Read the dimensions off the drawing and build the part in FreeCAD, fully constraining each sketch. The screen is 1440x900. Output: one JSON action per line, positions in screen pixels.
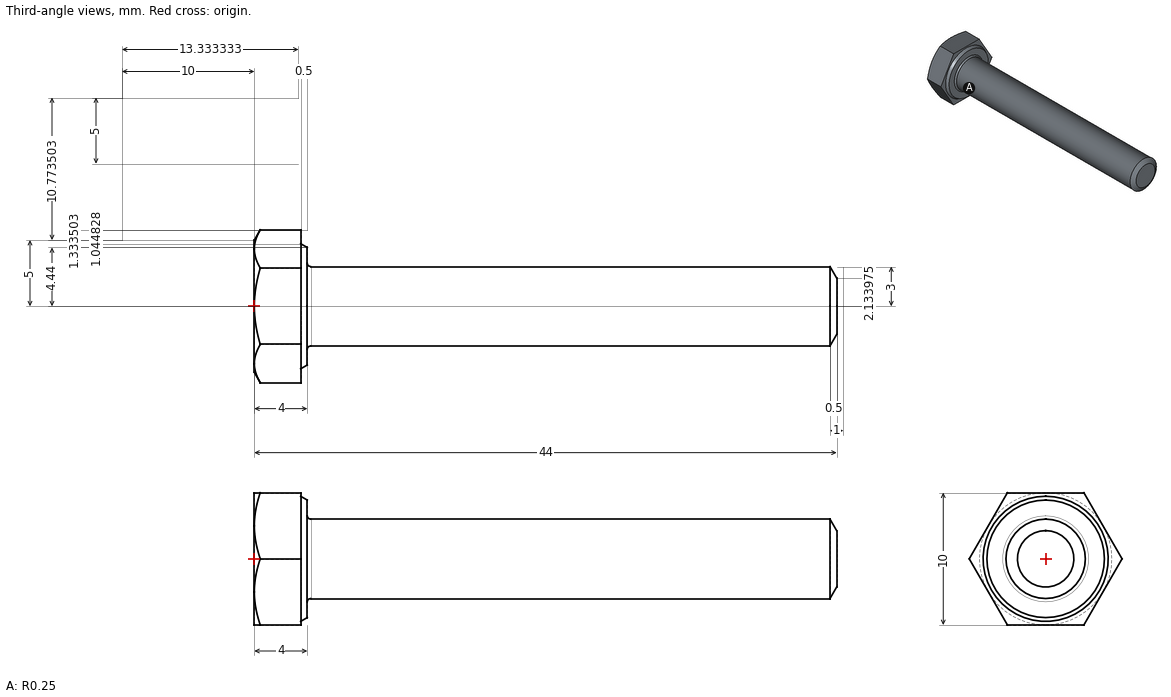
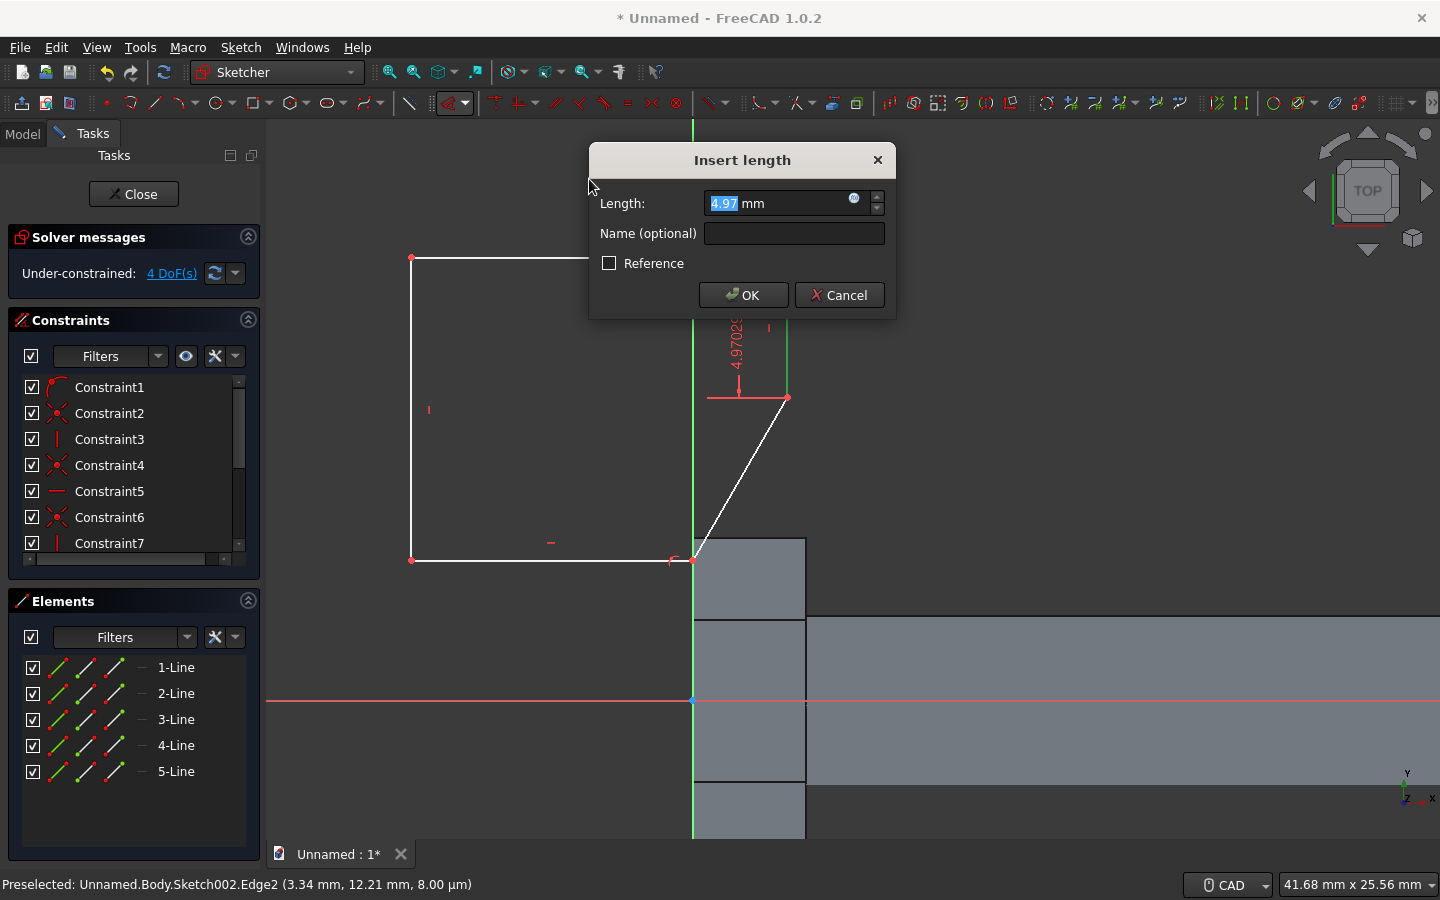
{"action": "type", "text": "5"}
{"action": "key", "text": "Return"}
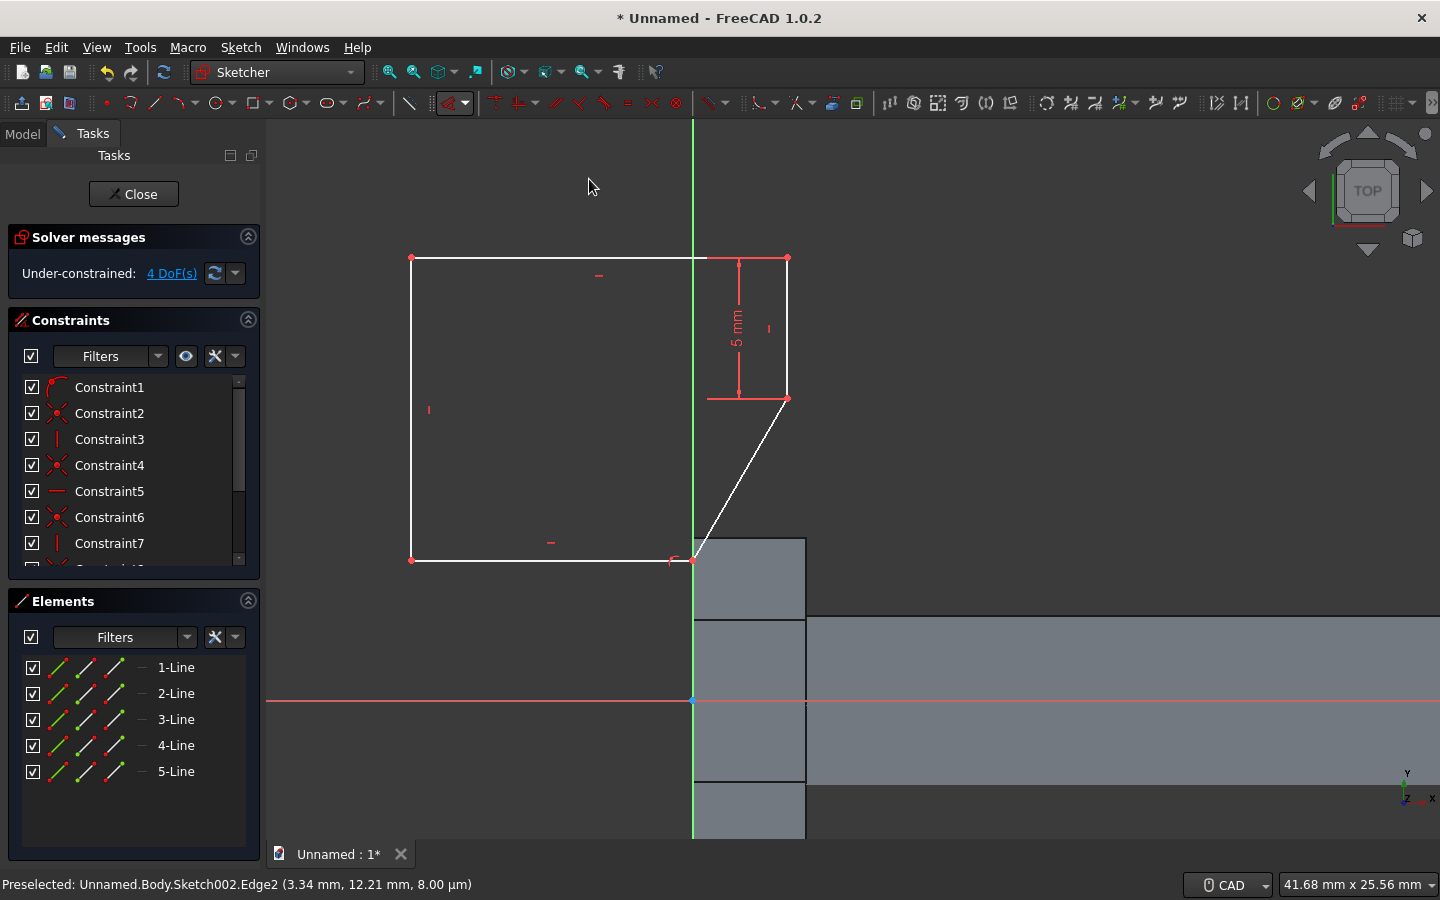
{"action": "left_click", "coordinate": [496, 561]}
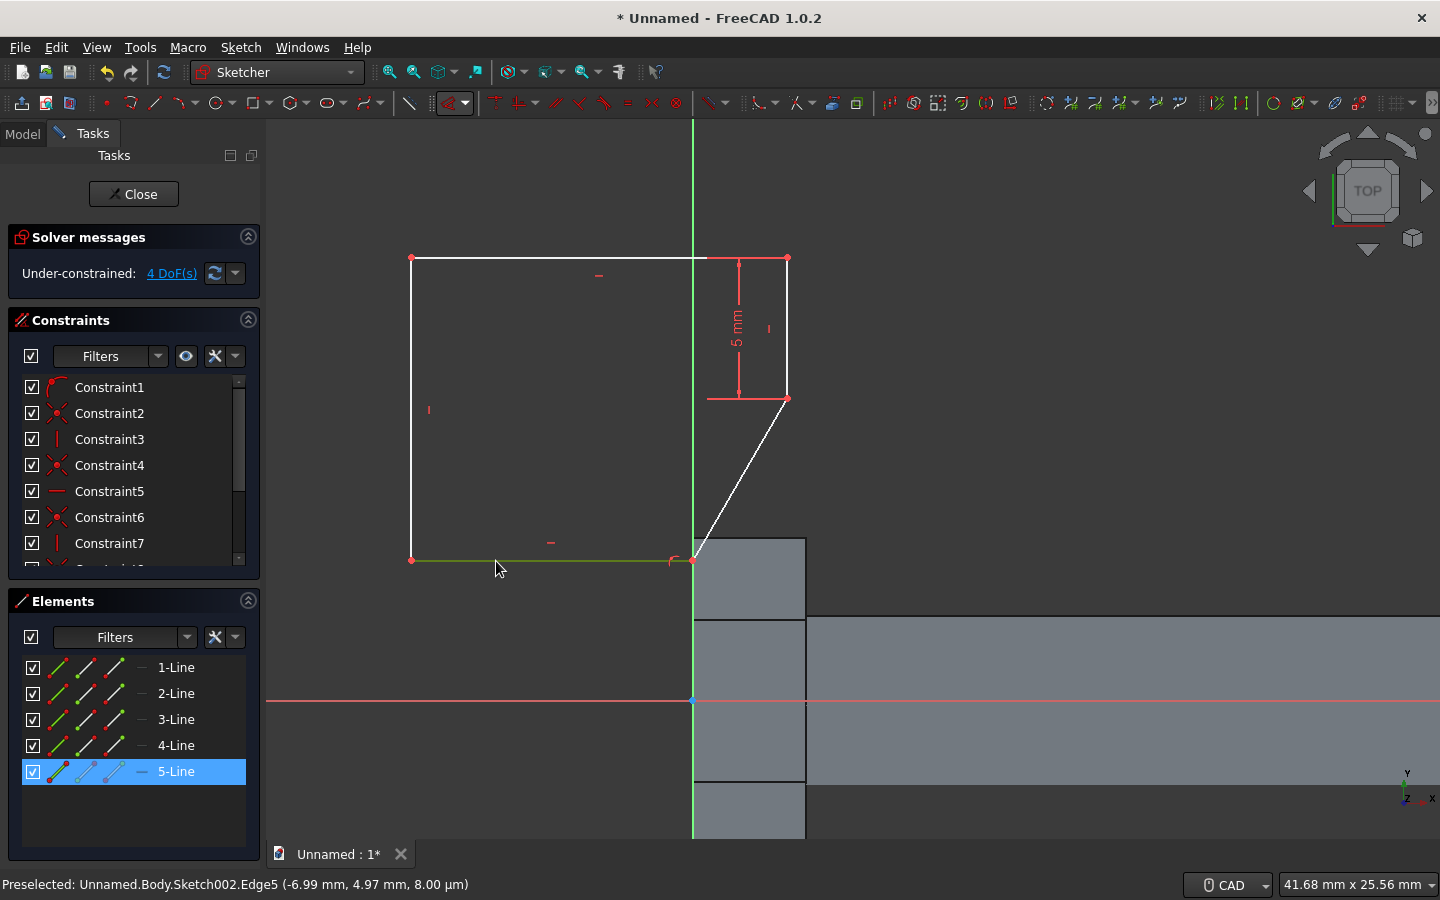
{"action": "left_click", "coordinate": [468, 104]}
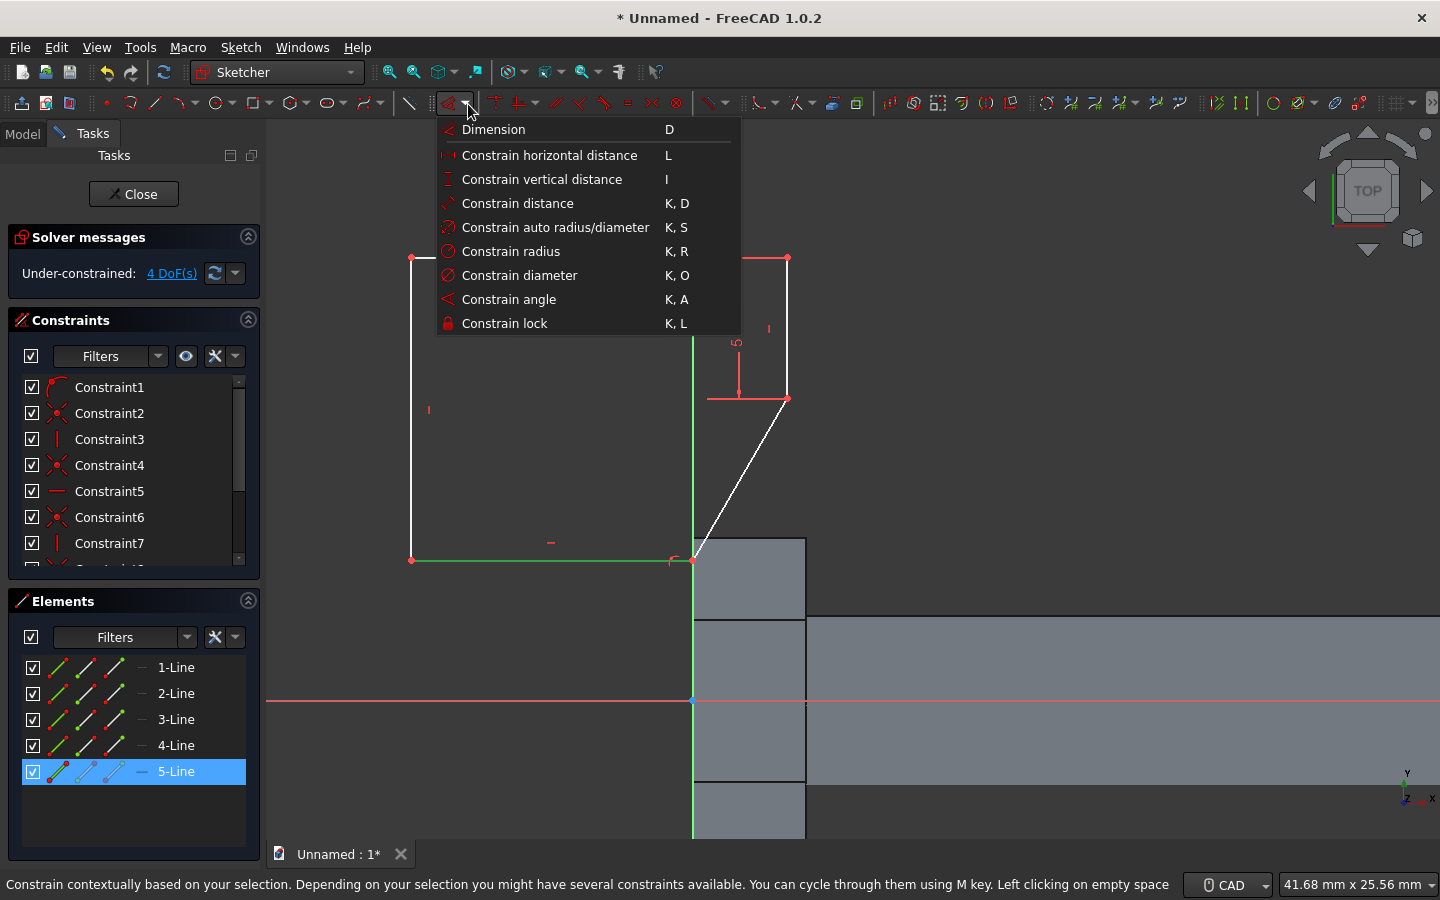
{"action": "left_click", "coordinate": [589, 155]}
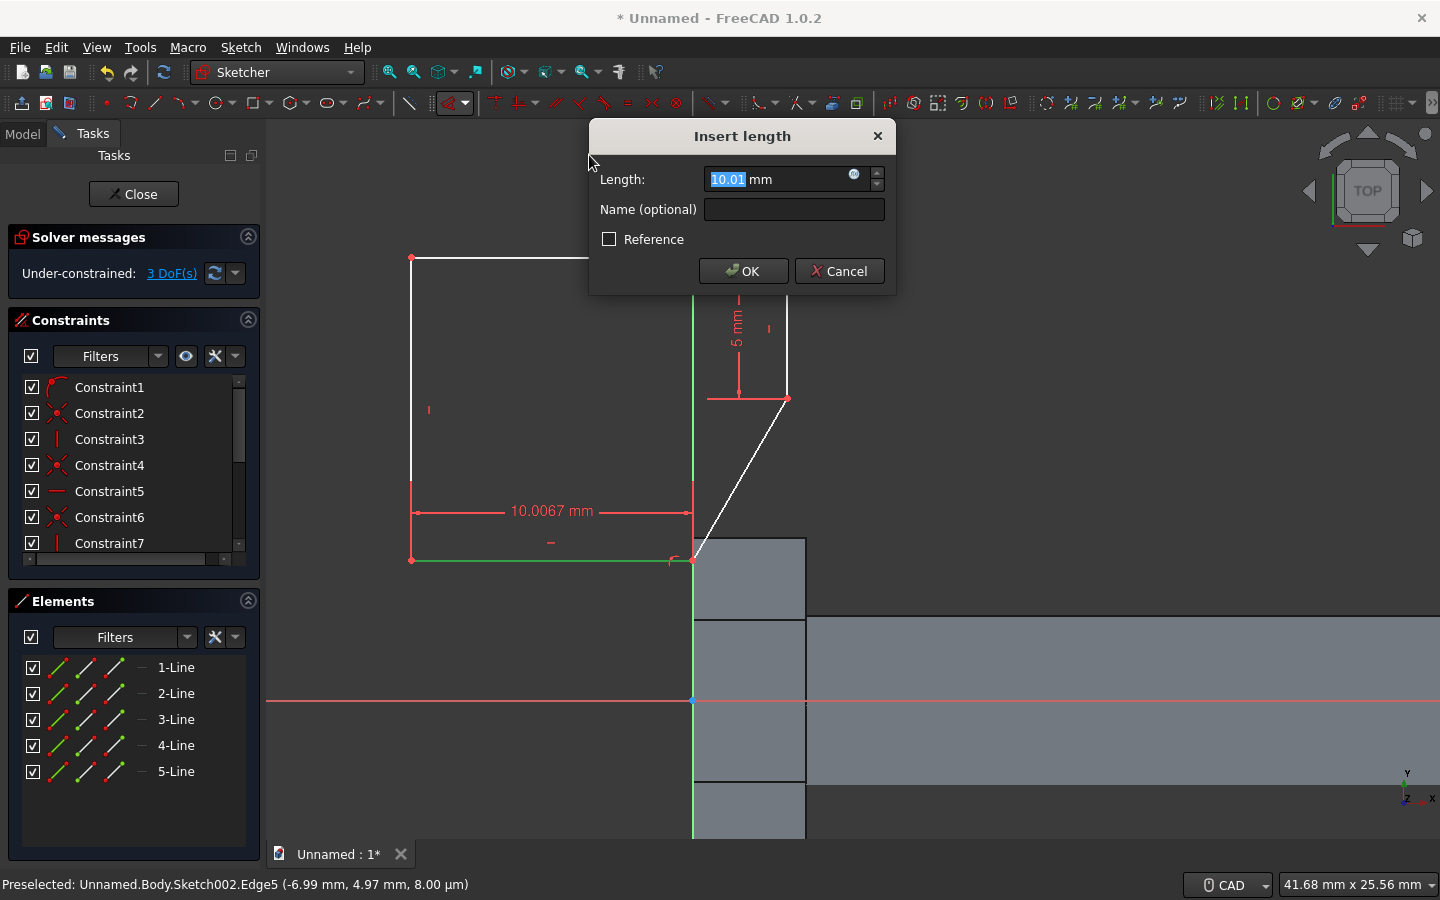
{"action": "type", "text": "10"}
{"action": "key", "text": "Return"}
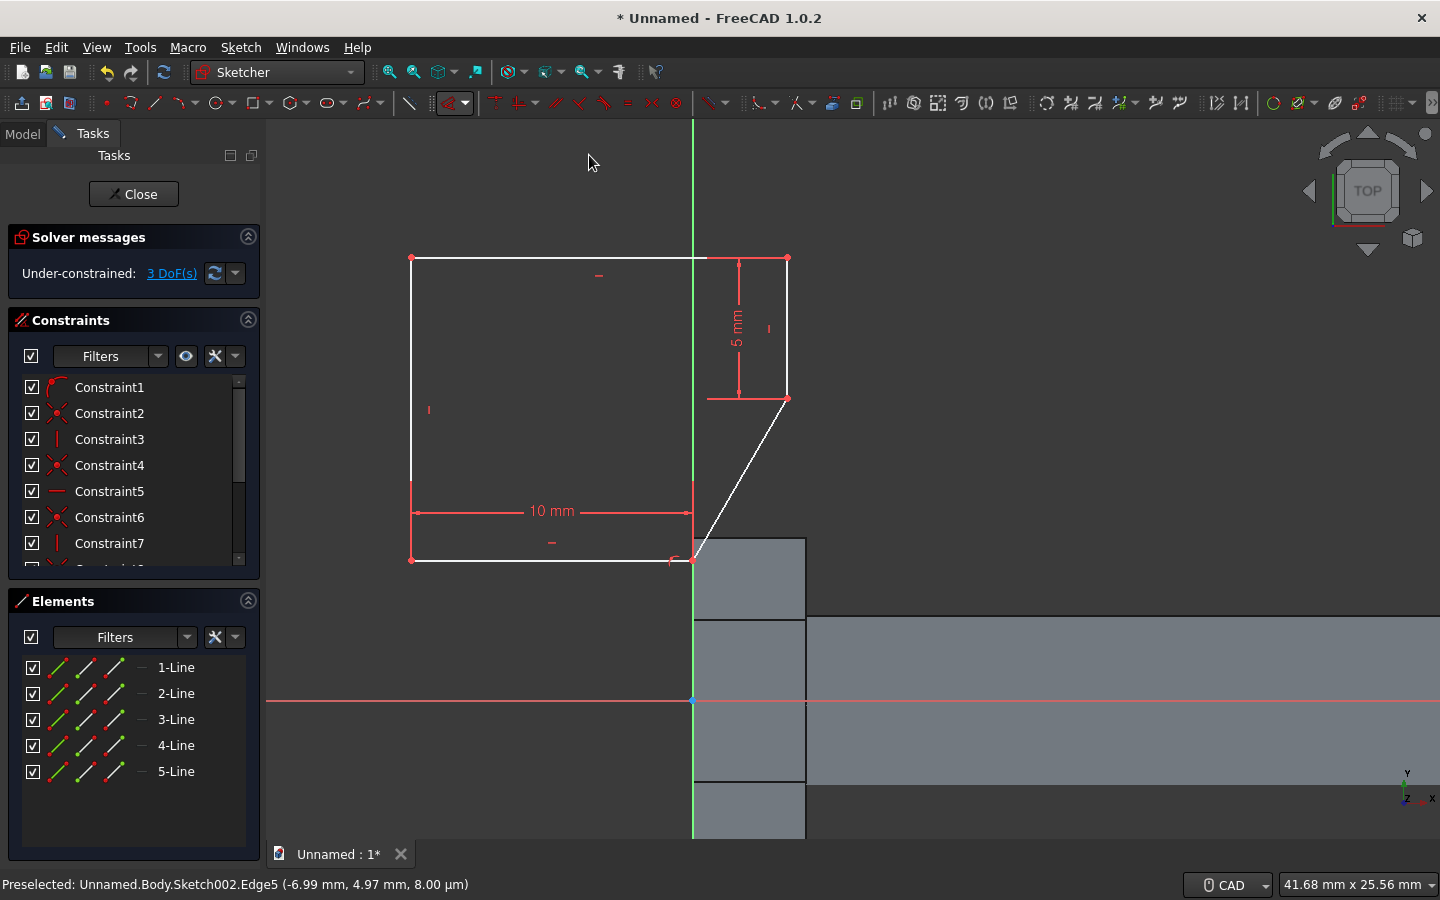
{"action": "left_click", "coordinate": [693, 561]}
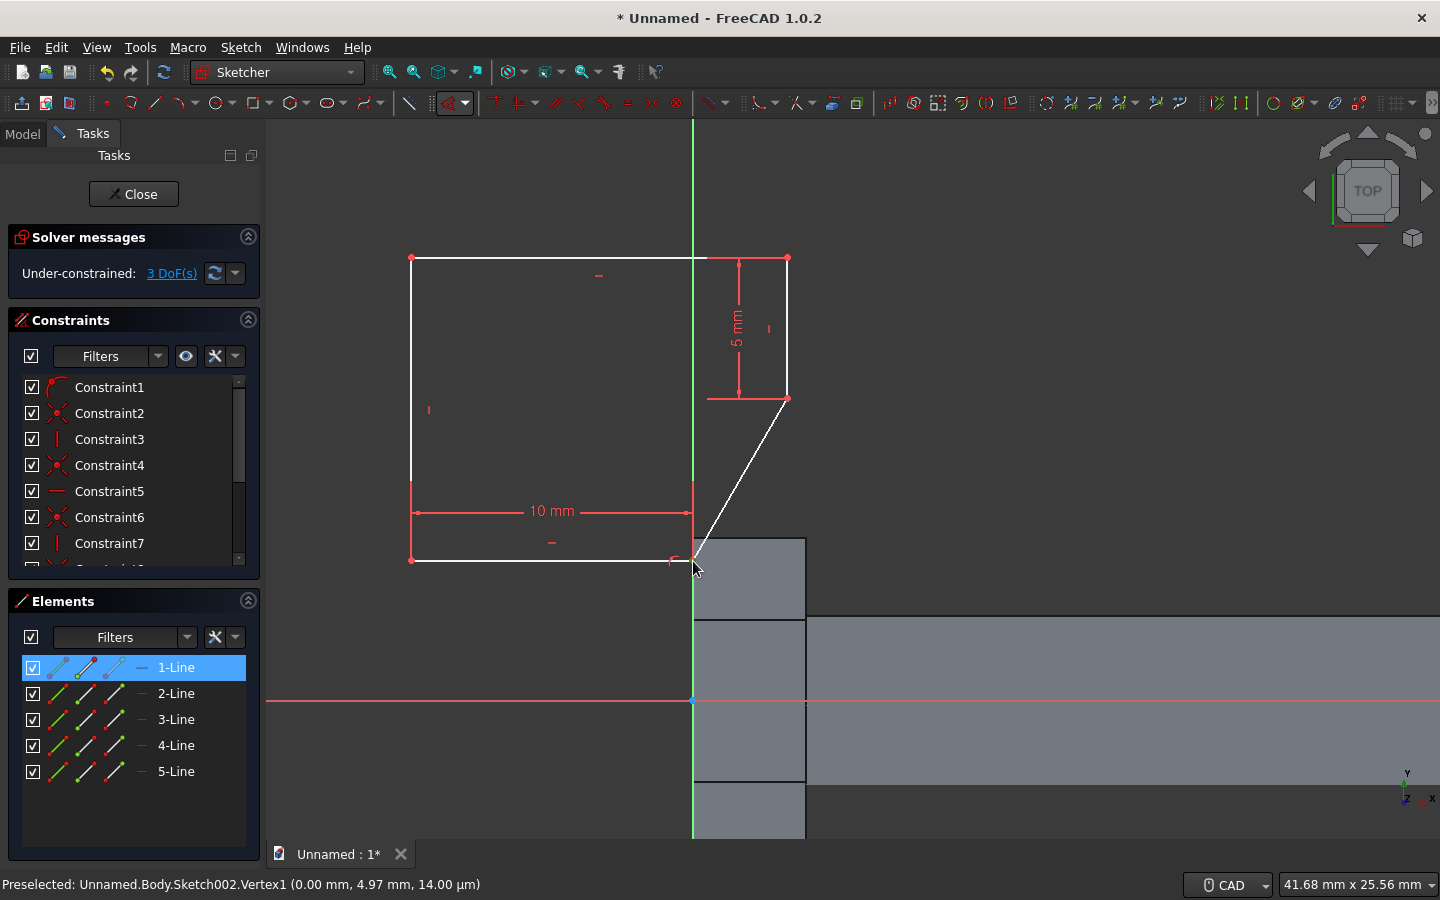
{"action": "left_click", "coordinate": [468, 104]}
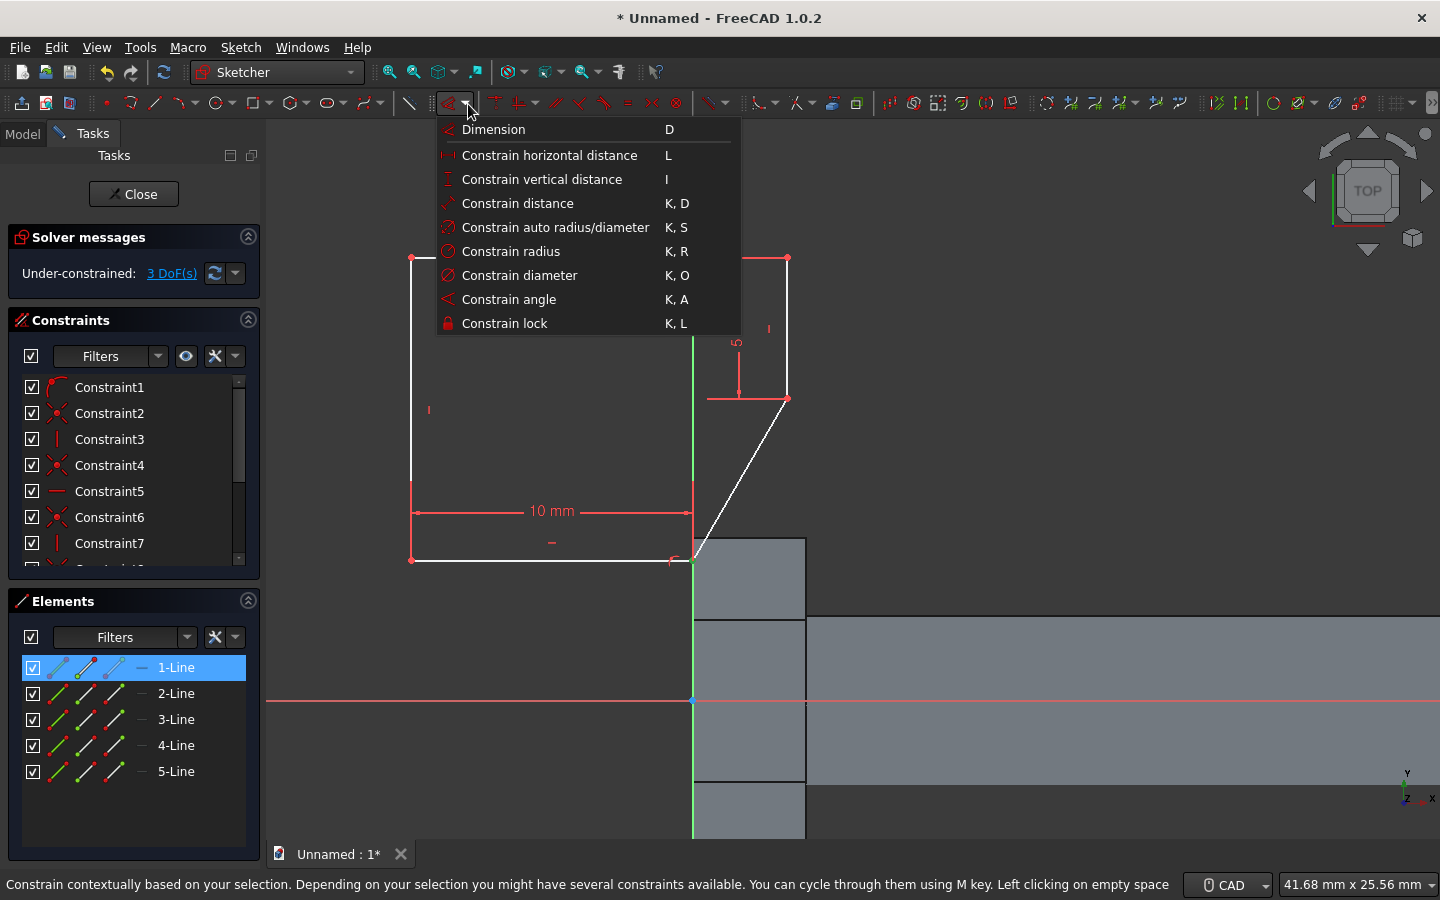
{"action": "left_click", "coordinate": [589, 179]}